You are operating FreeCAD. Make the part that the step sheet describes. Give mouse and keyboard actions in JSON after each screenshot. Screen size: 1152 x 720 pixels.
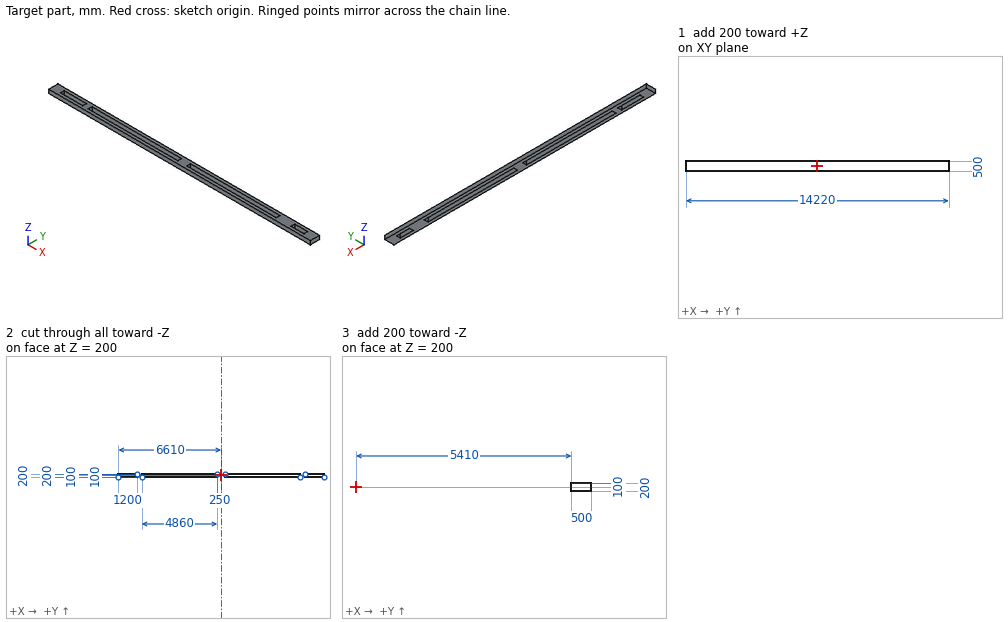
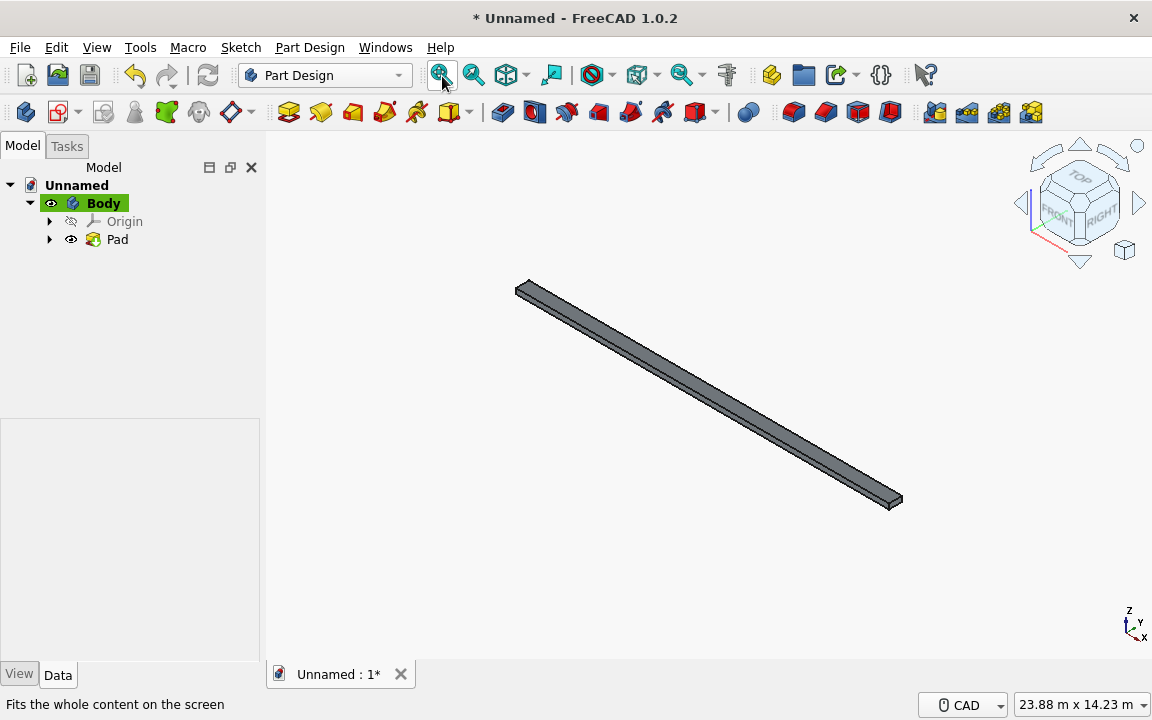
{"action": "left_click", "coordinate": [442, 76]}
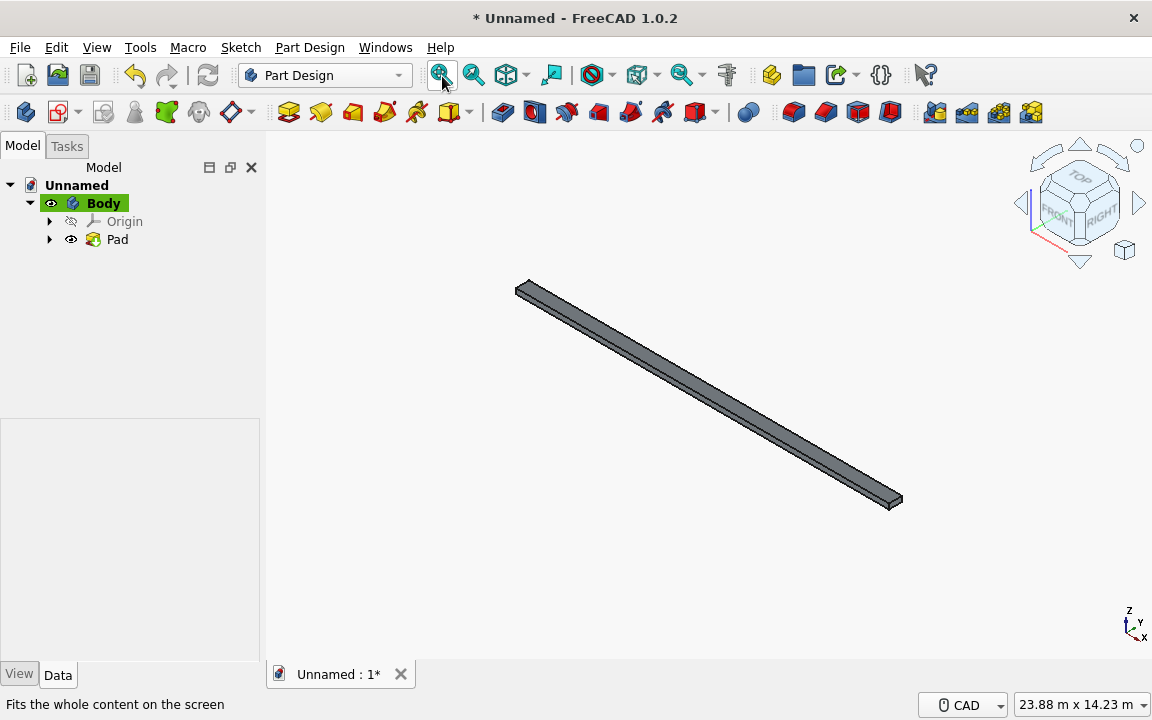
{"action": "key", "text": "2"}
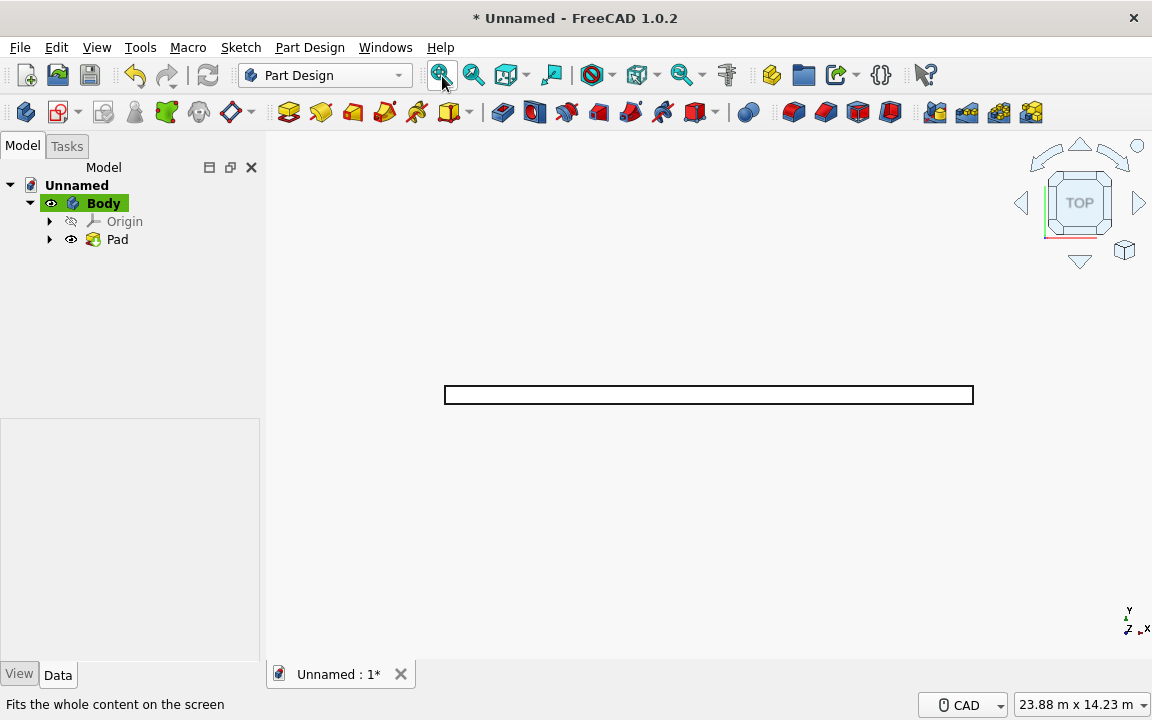
{"action": "left_click", "coordinate": [935, 394]}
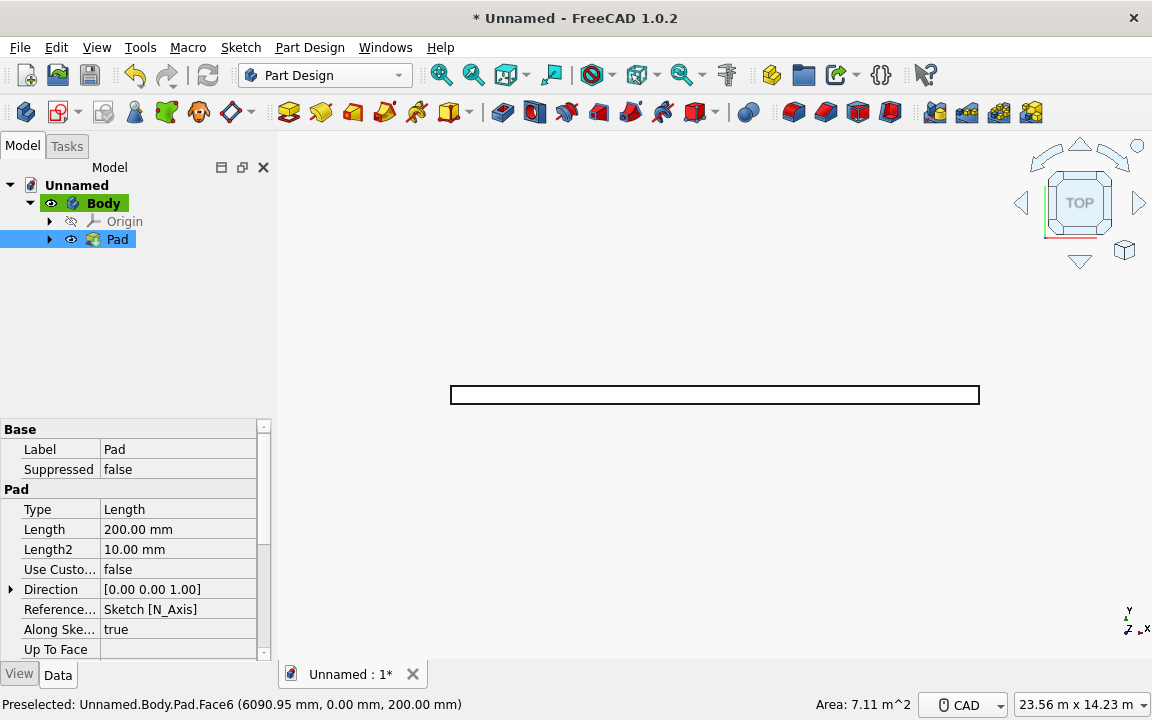
{"action": "left_click", "coordinate": [58, 112]}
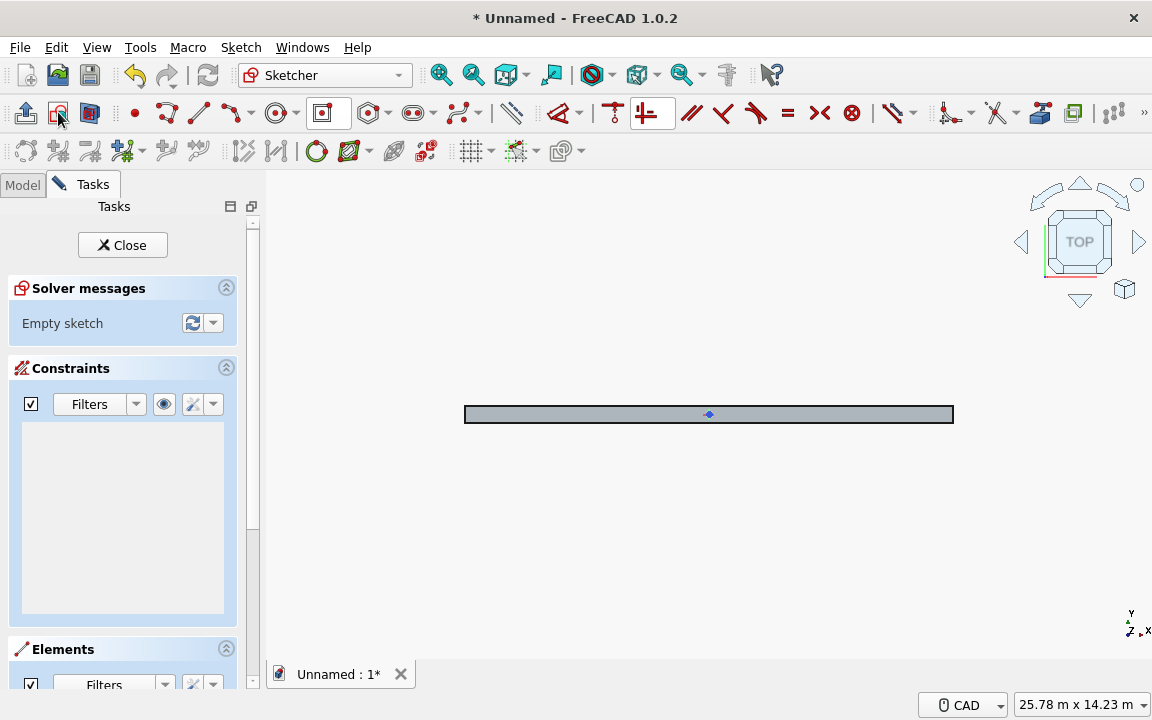
{"action": "left_click", "coordinate": [346, 114]}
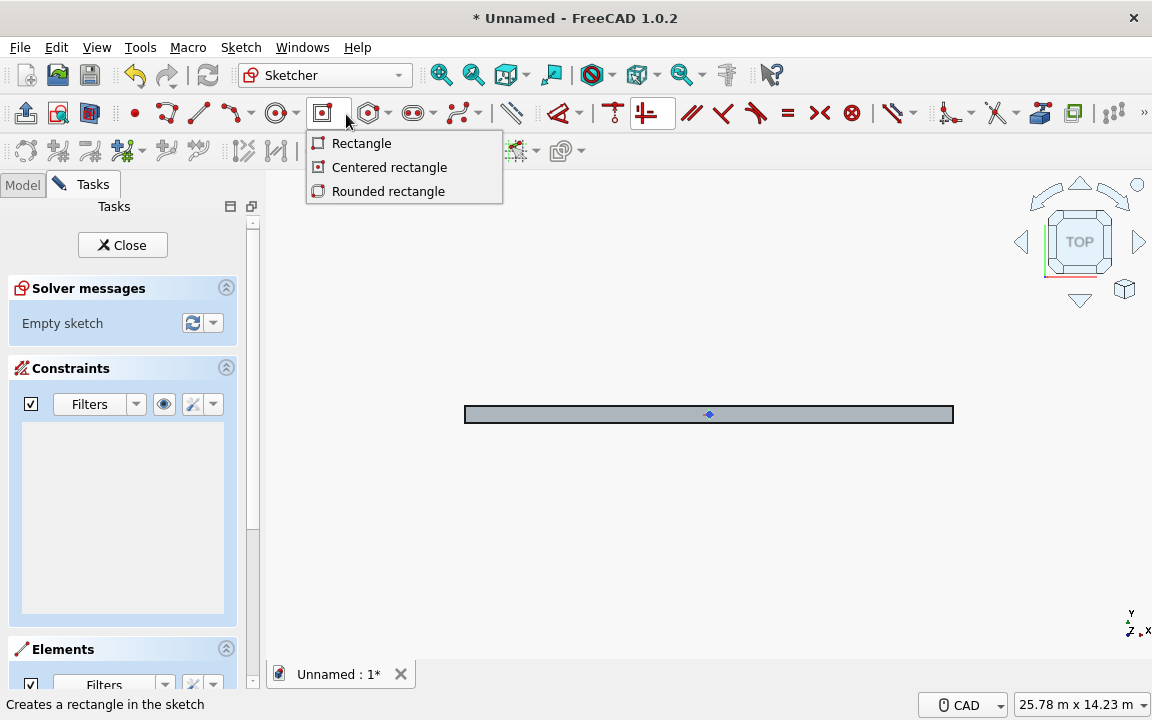
{"action": "left_click", "coordinate": [404, 143]}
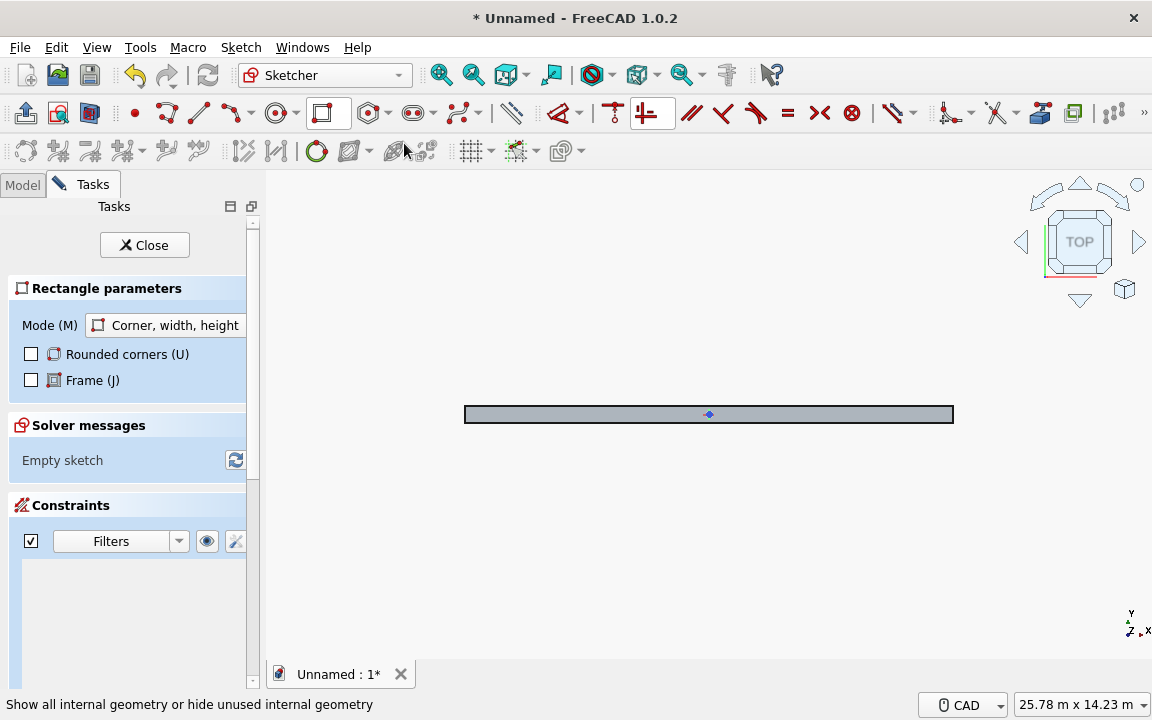
{"action": "scroll", "coordinate": [482, 411], "scroll_direction": "up", "scroll_amount": 8}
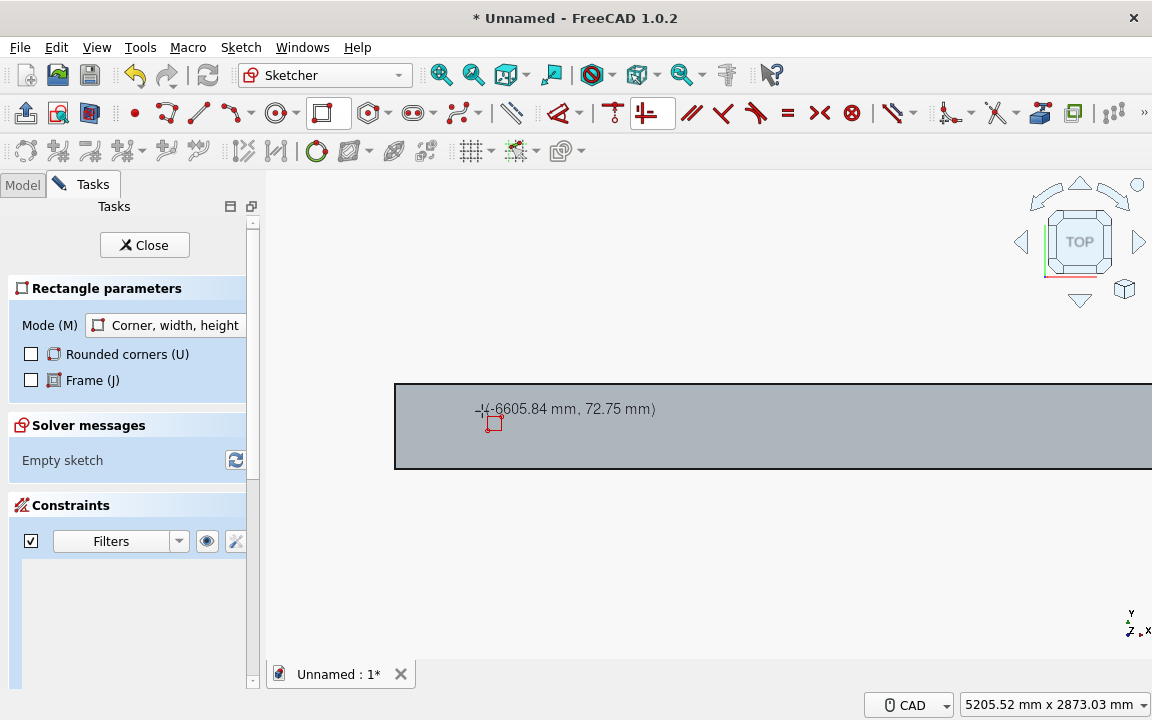
{"action": "left_click", "coordinate": [480, 409]}
{"action": "mouse_move", "coordinate": [685, 443]}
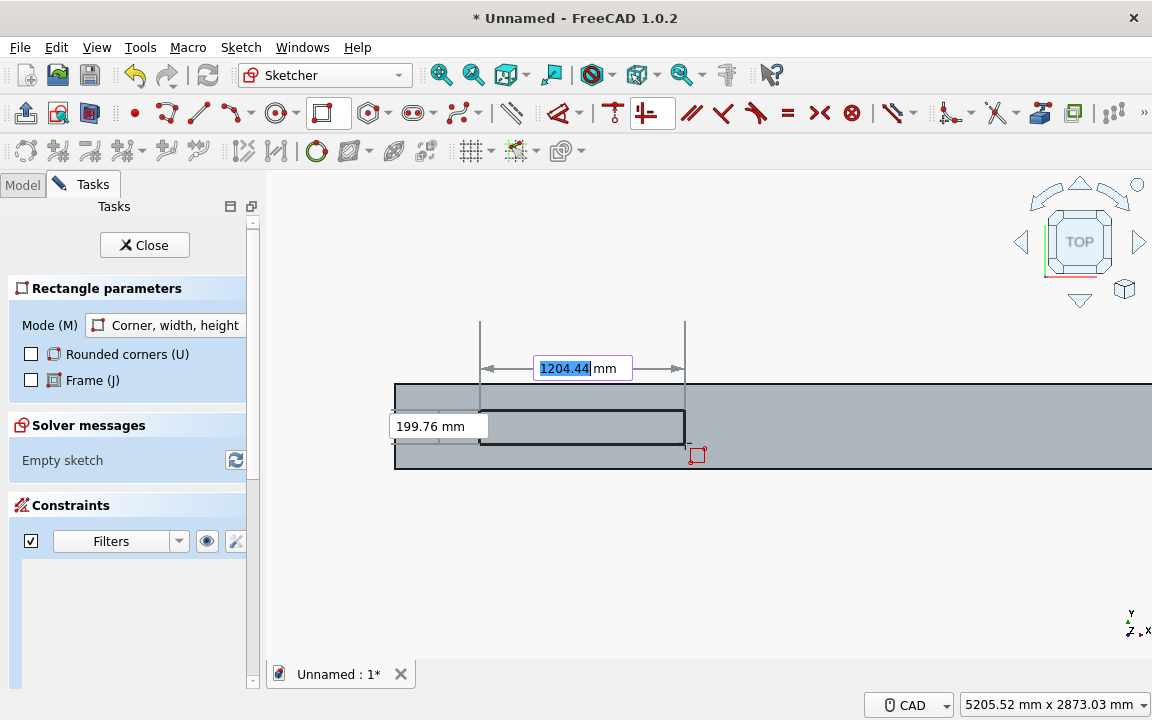
{"action": "type", "text": "1200"}
{"action": "key", "text": "Tab"}
{"action": "type", "text": "200"}
{"action": "key", "text": "Return"}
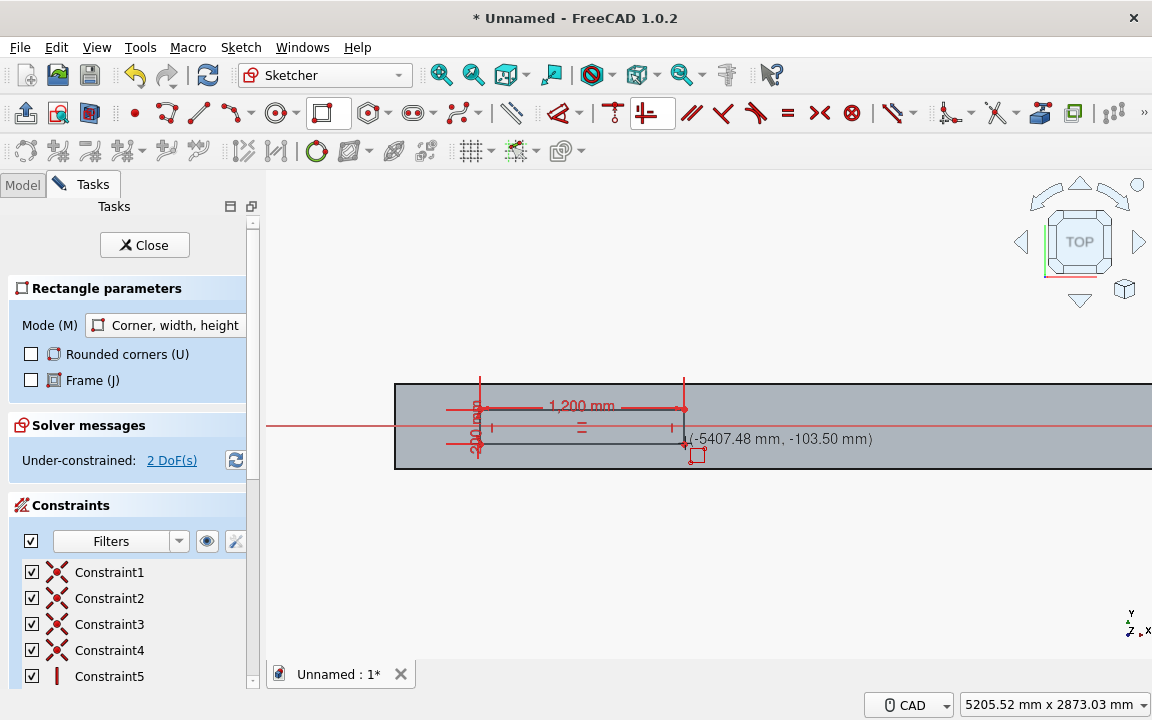
{"action": "left_click", "coordinate": [736, 409]}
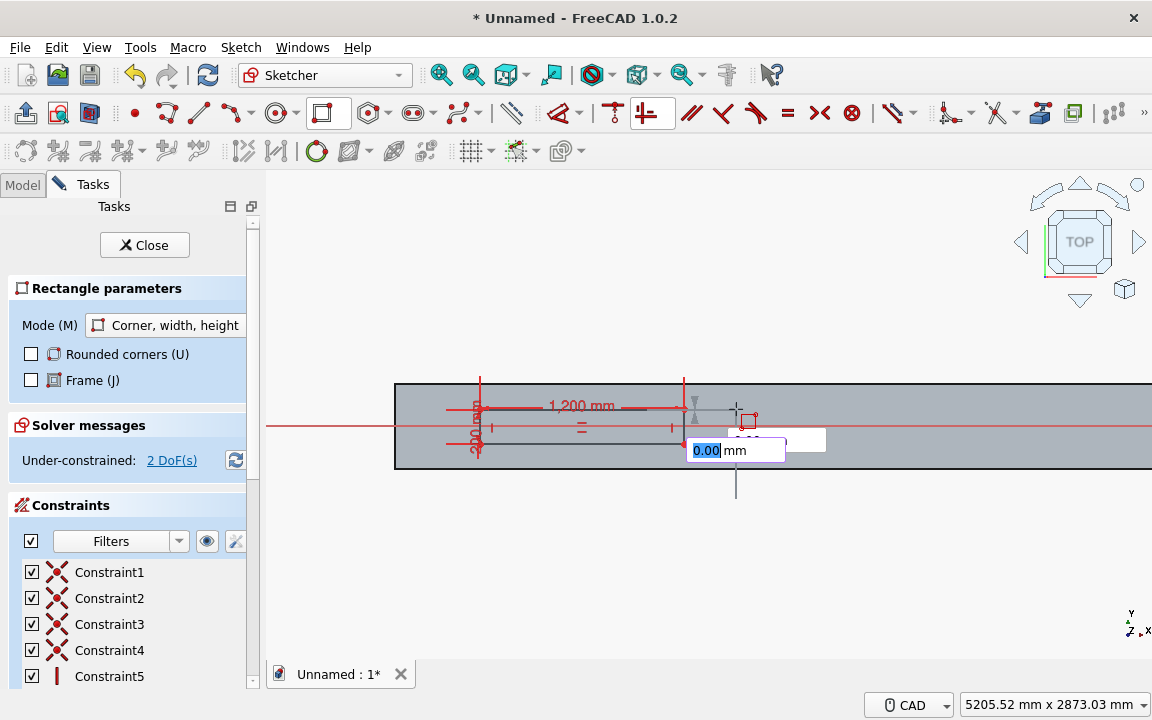
{"action": "scroll", "coordinate": [396, 411], "scroll_direction": "down", "scroll_amount": 8}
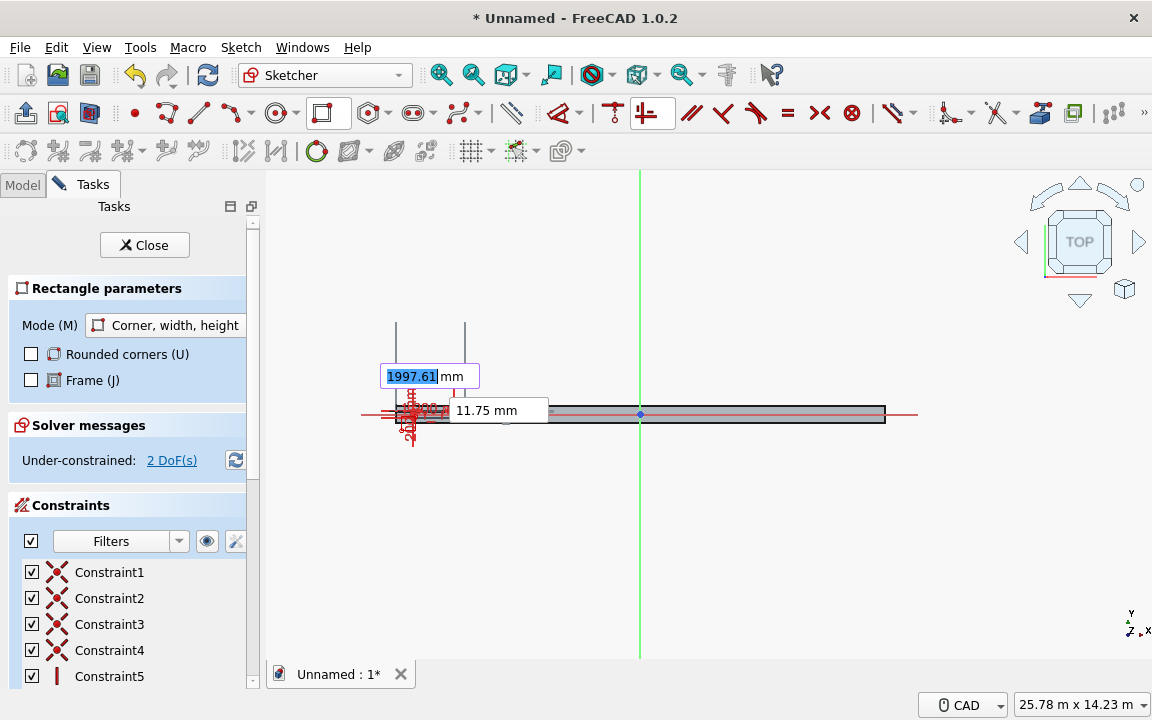
{"action": "scroll", "coordinate": [632, 418], "scroll_direction": "up", "scroll_amount": 8}